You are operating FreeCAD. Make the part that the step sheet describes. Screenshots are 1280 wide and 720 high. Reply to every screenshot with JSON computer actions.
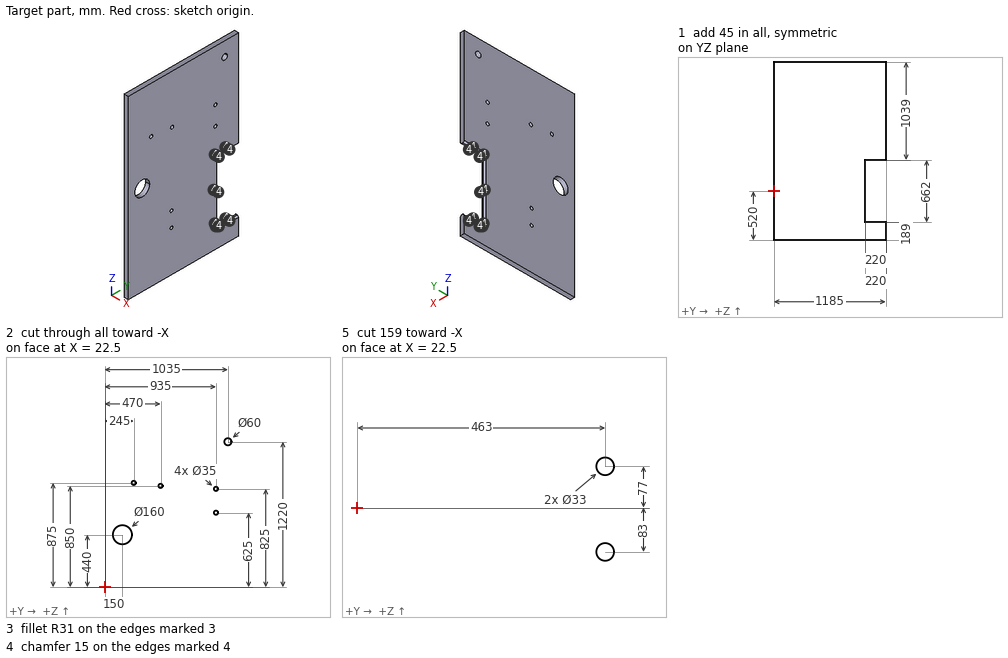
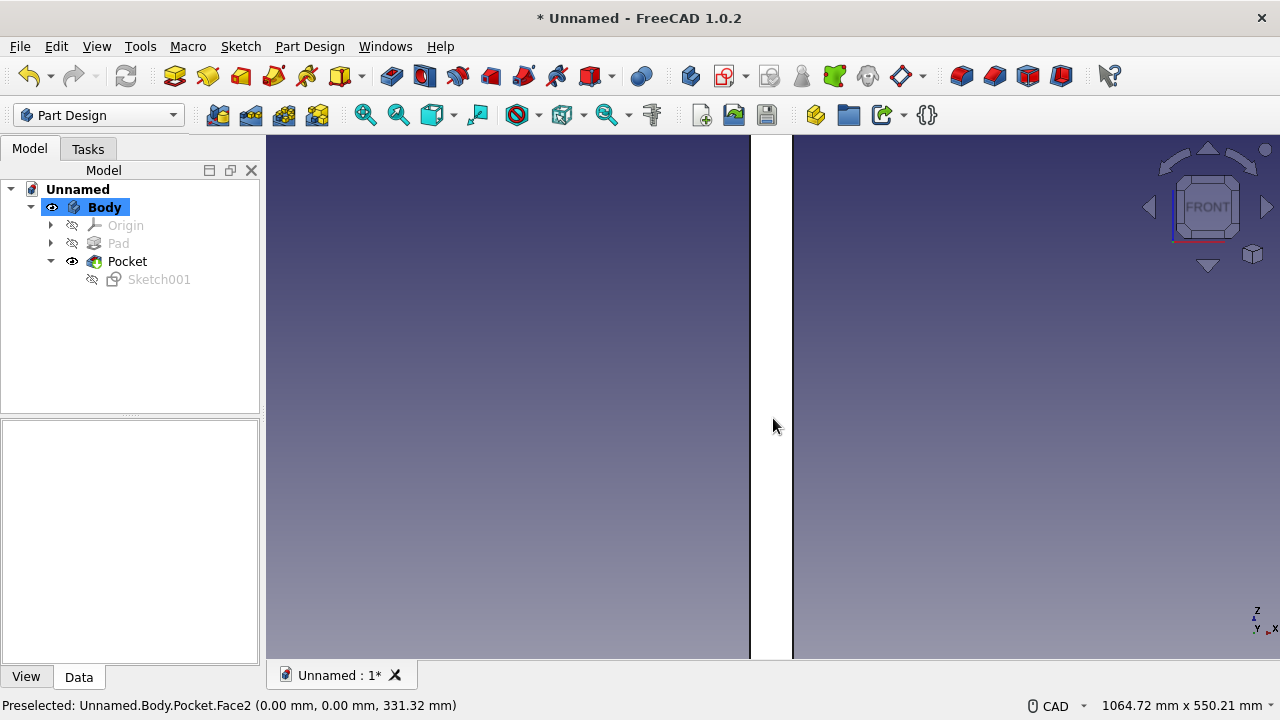
{"action": "left_click", "coordinate": [366, 116]}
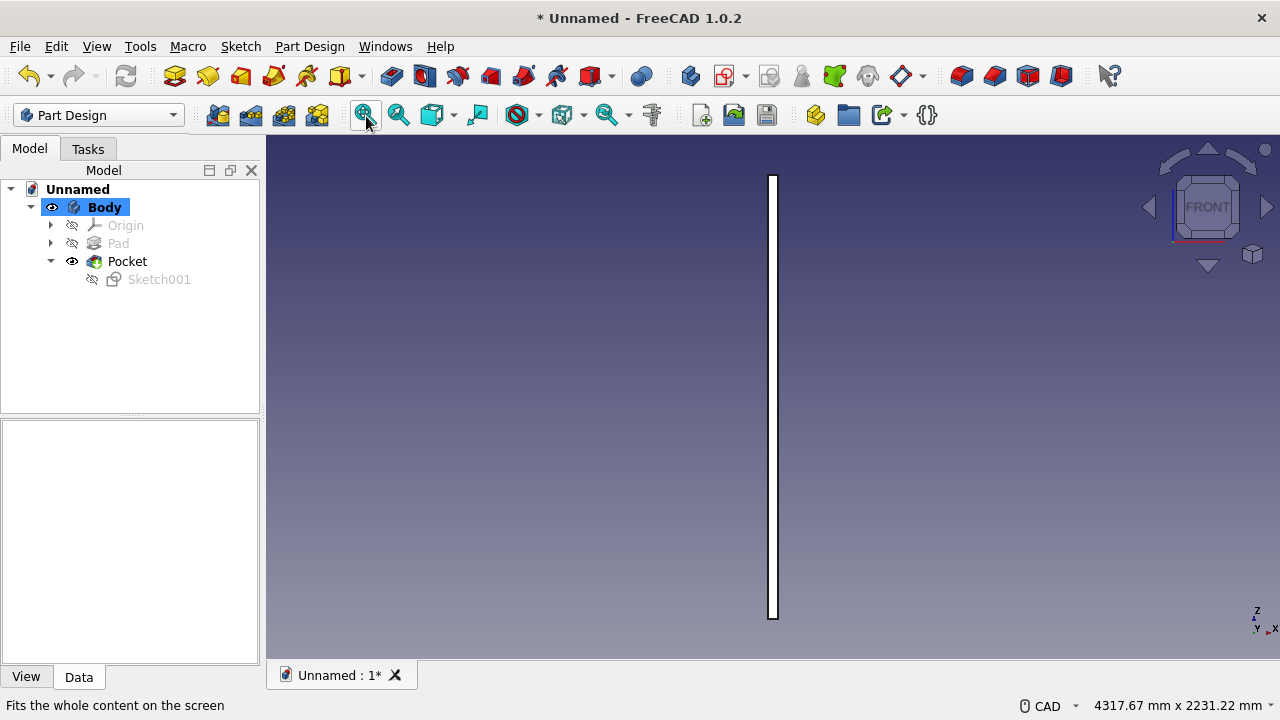
{"action": "key", "text": "3"}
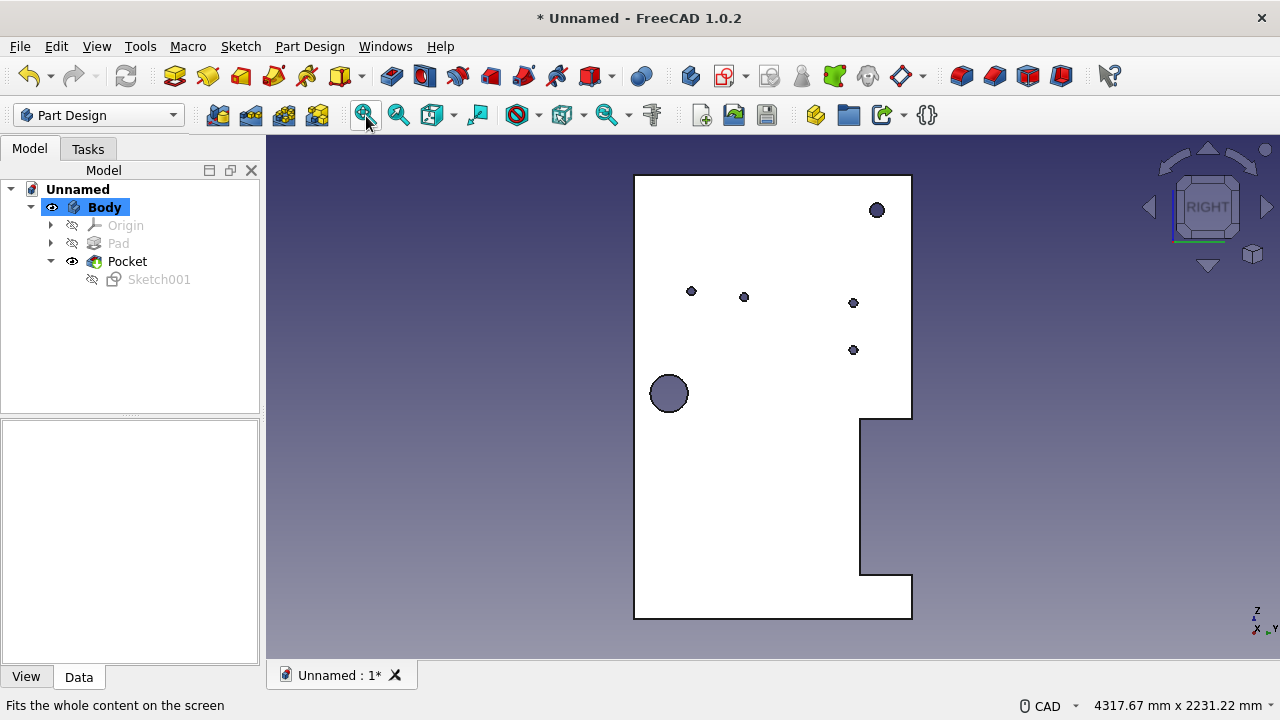
{"action": "scroll", "coordinate": [860, 418], "scroll_direction": "up", "scroll_amount": 7}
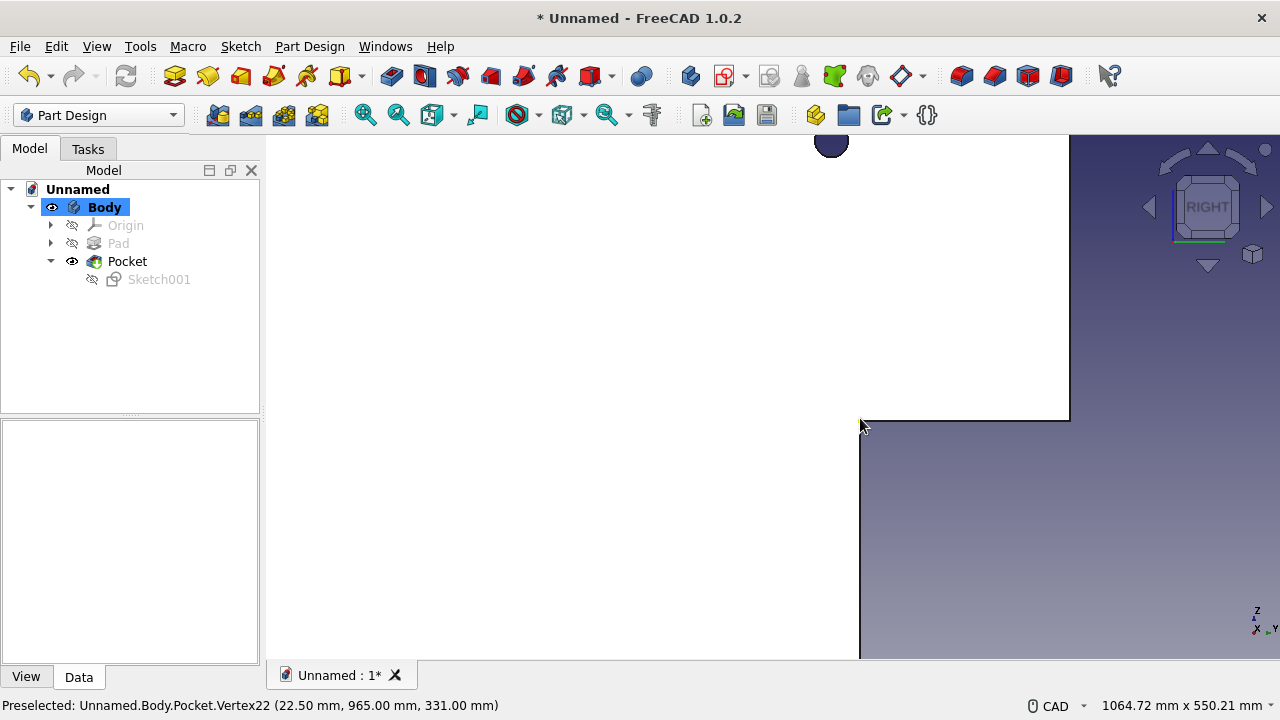
{"action": "left_click", "coordinate": [366, 116]}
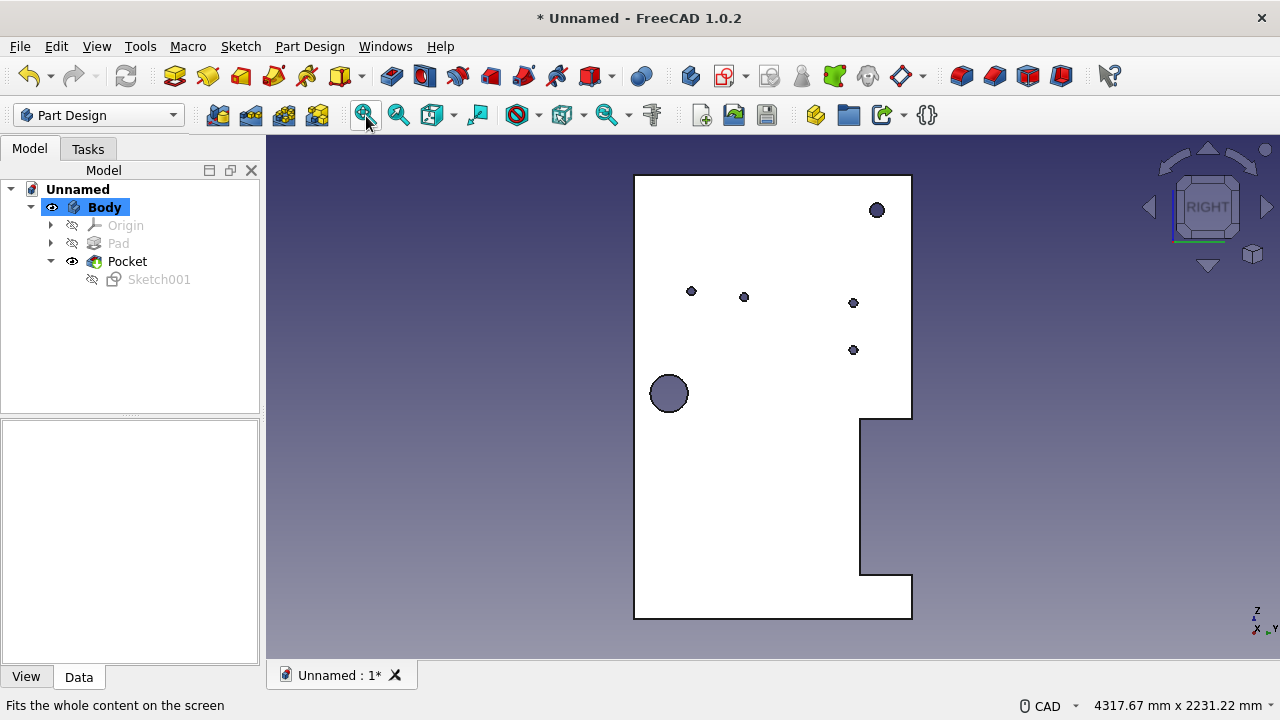
{"action": "key", "text": "5"}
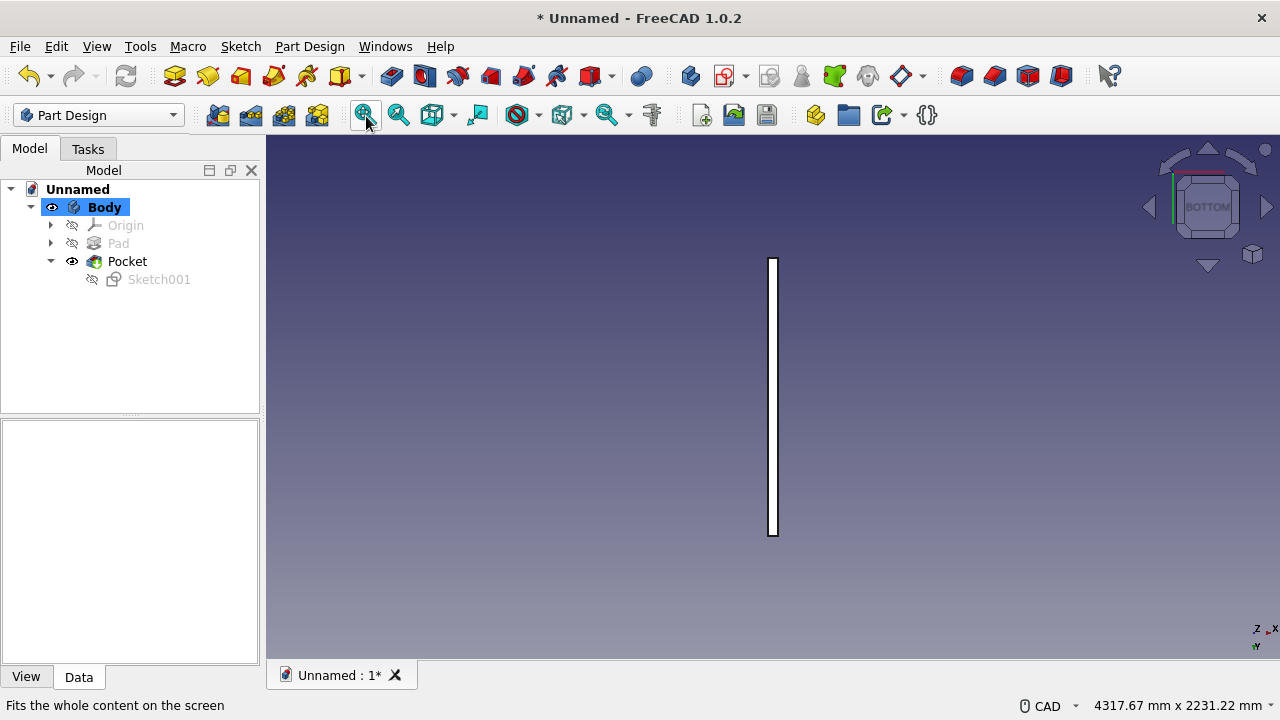
{"action": "scroll", "coordinate": [773, 483], "scroll_direction": "up", "scroll_amount": 7}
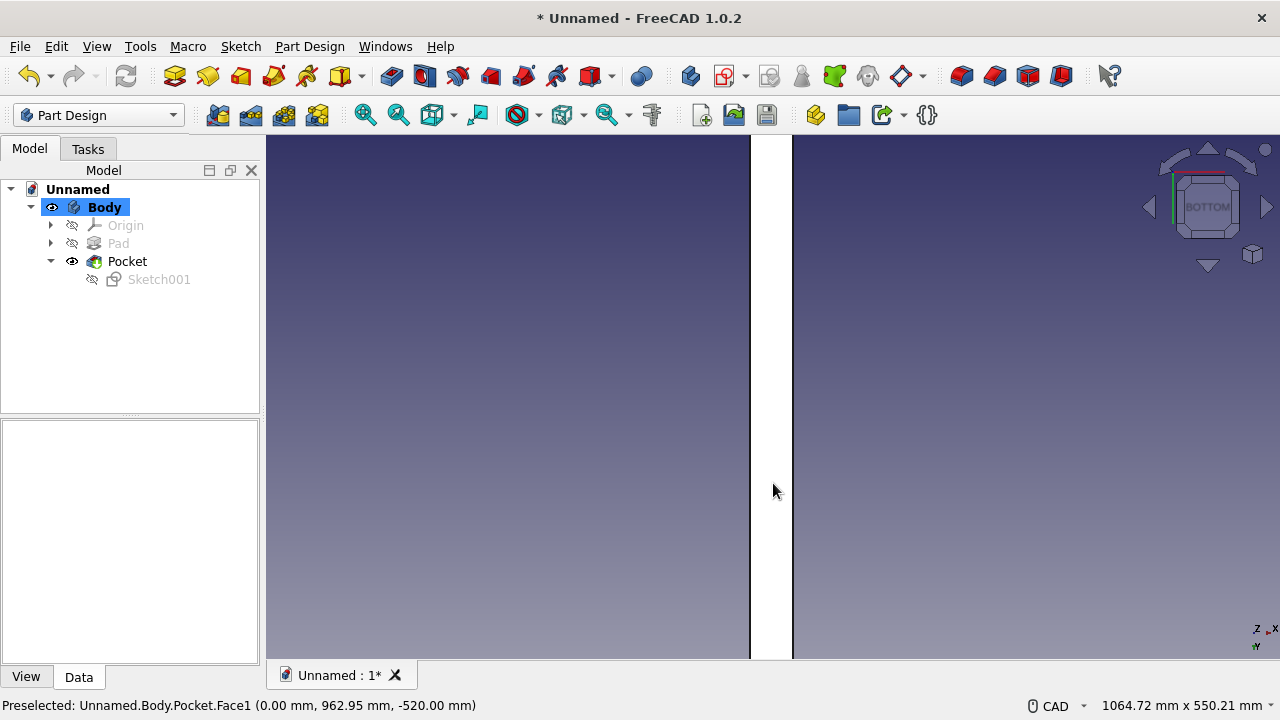
{"action": "left_click", "coordinate": [366, 116]}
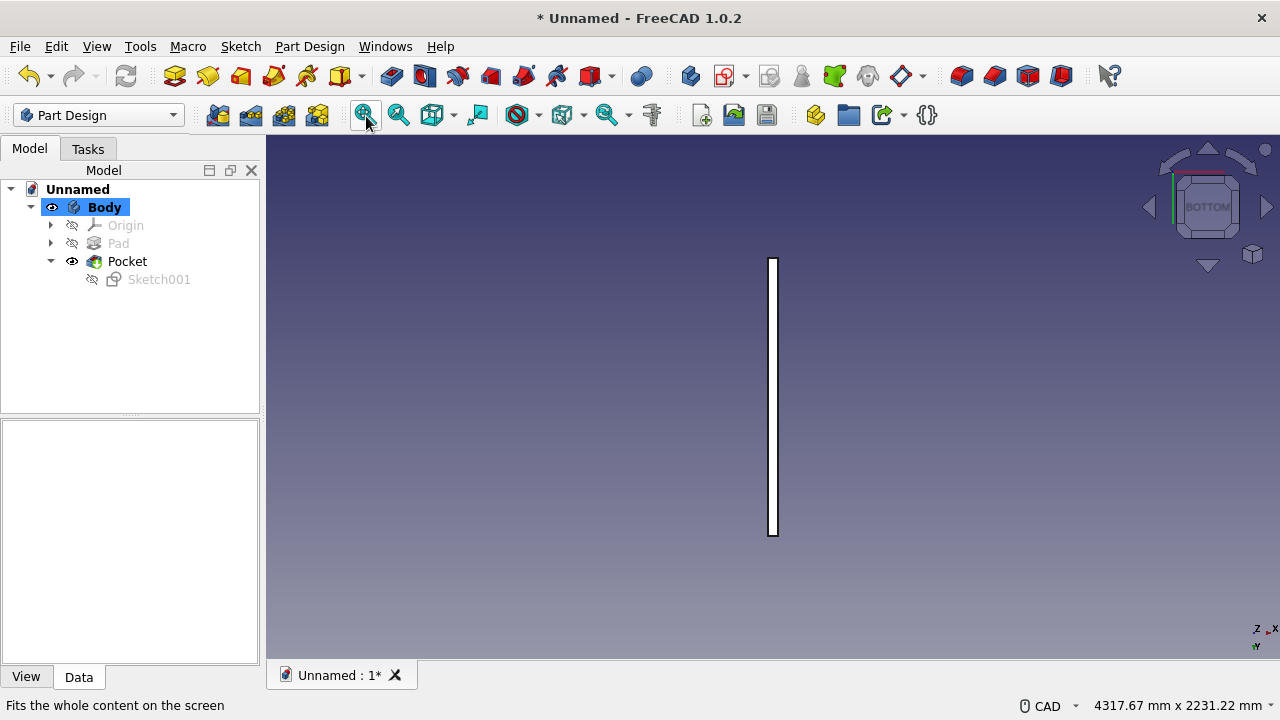
{"action": "key", "text": "4"}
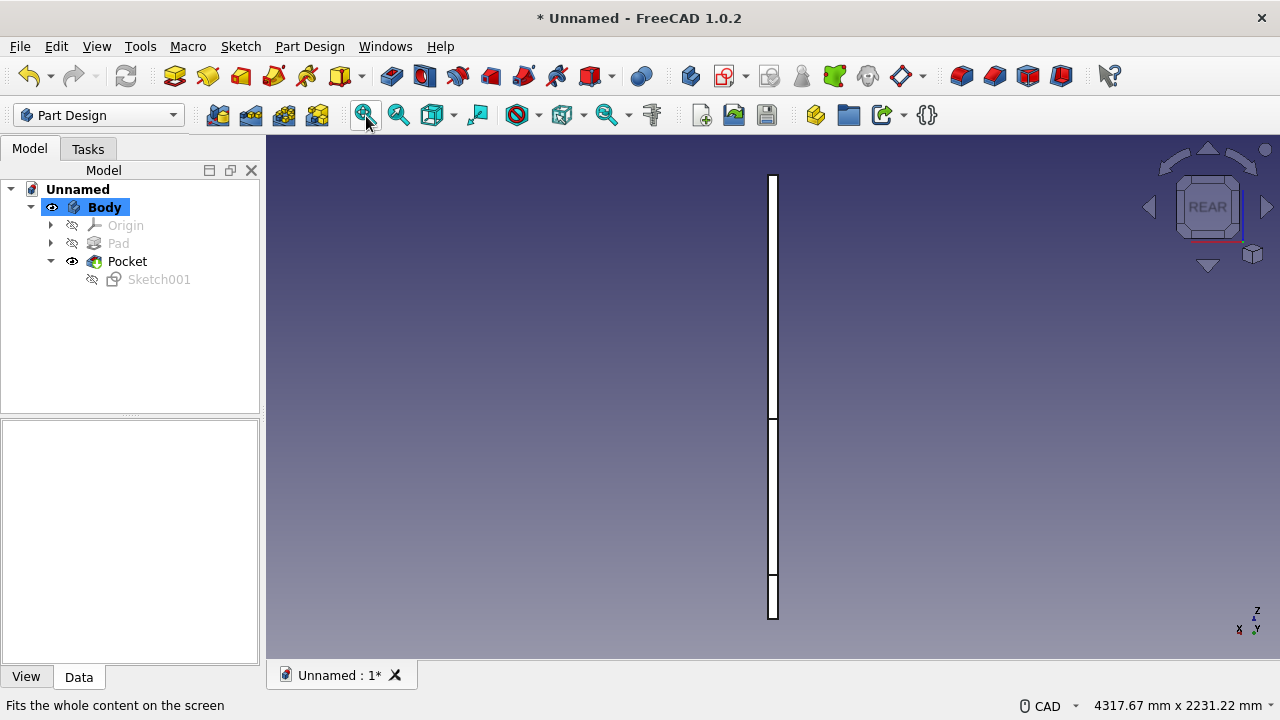
{"action": "scroll", "coordinate": [773, 418], "scroll_direction": "up", "scroll_amount": 7}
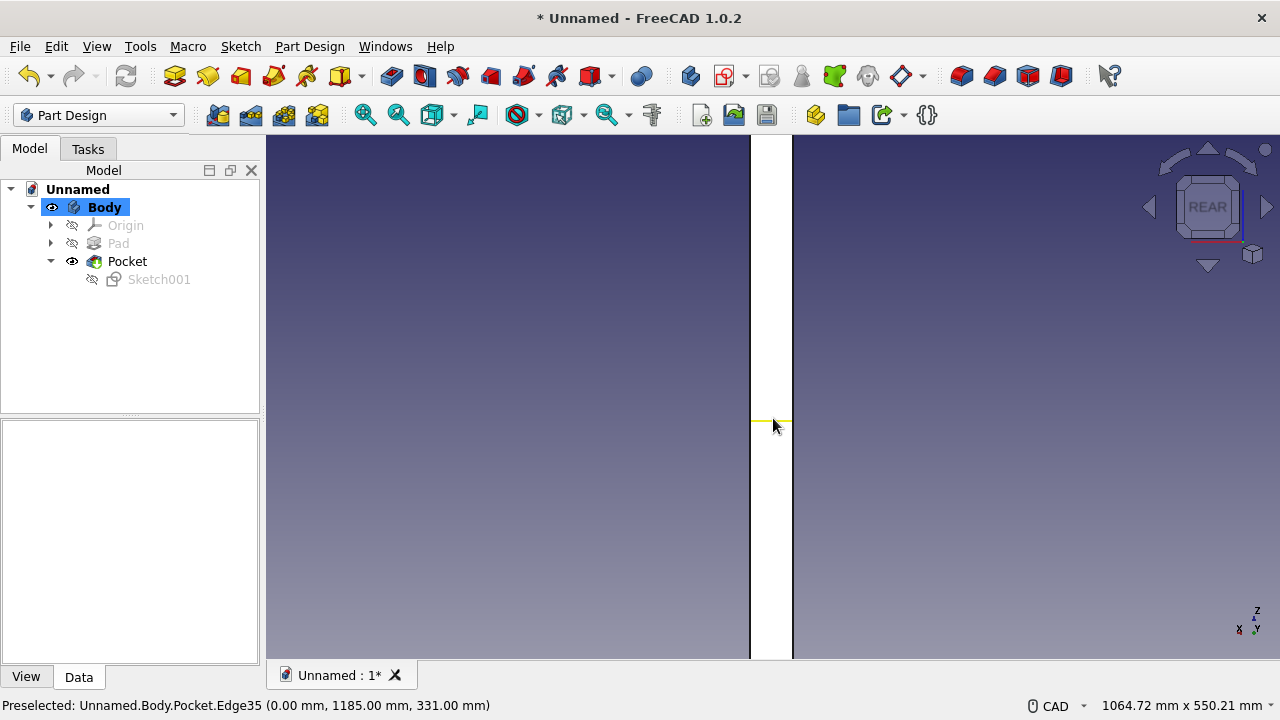
{"action": "left_click", "coordinate": [366, 116]}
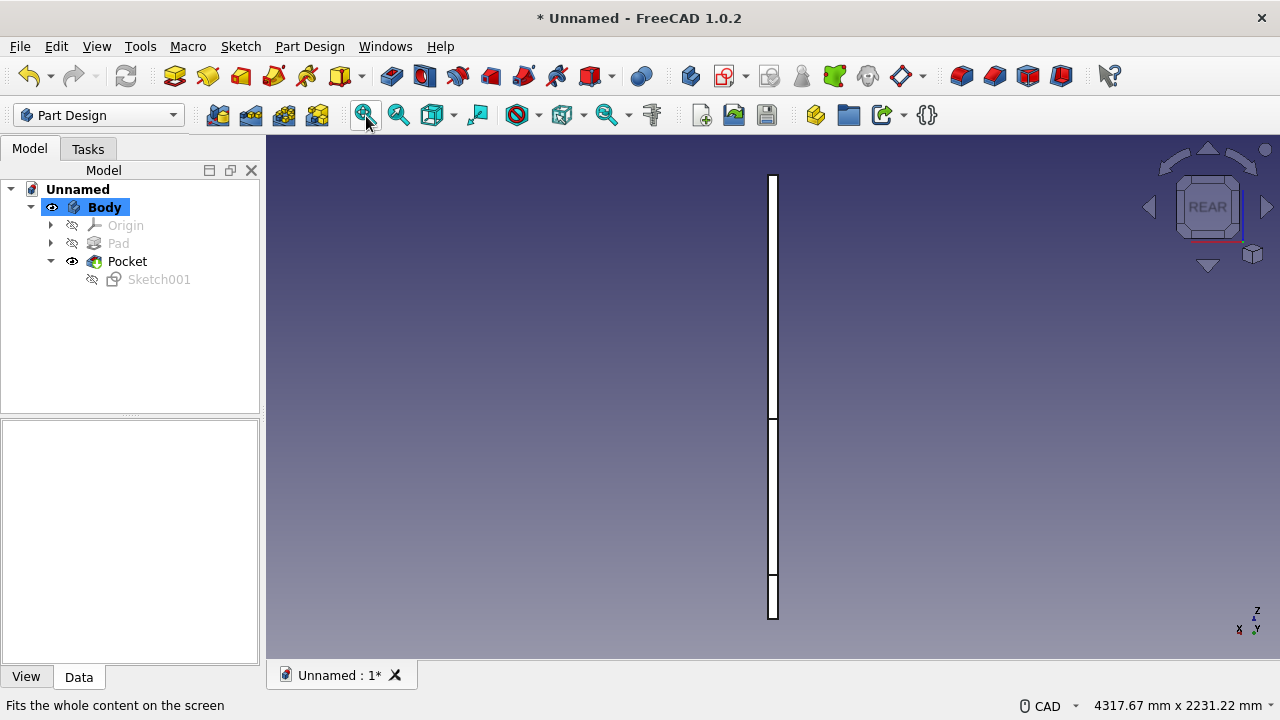
{"action": "key", "text": "6"}